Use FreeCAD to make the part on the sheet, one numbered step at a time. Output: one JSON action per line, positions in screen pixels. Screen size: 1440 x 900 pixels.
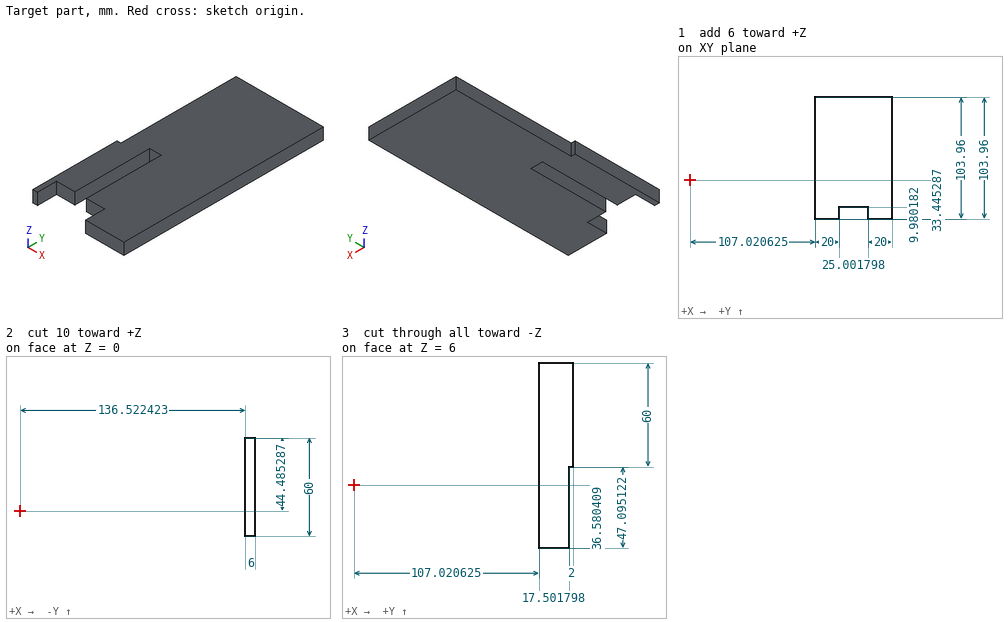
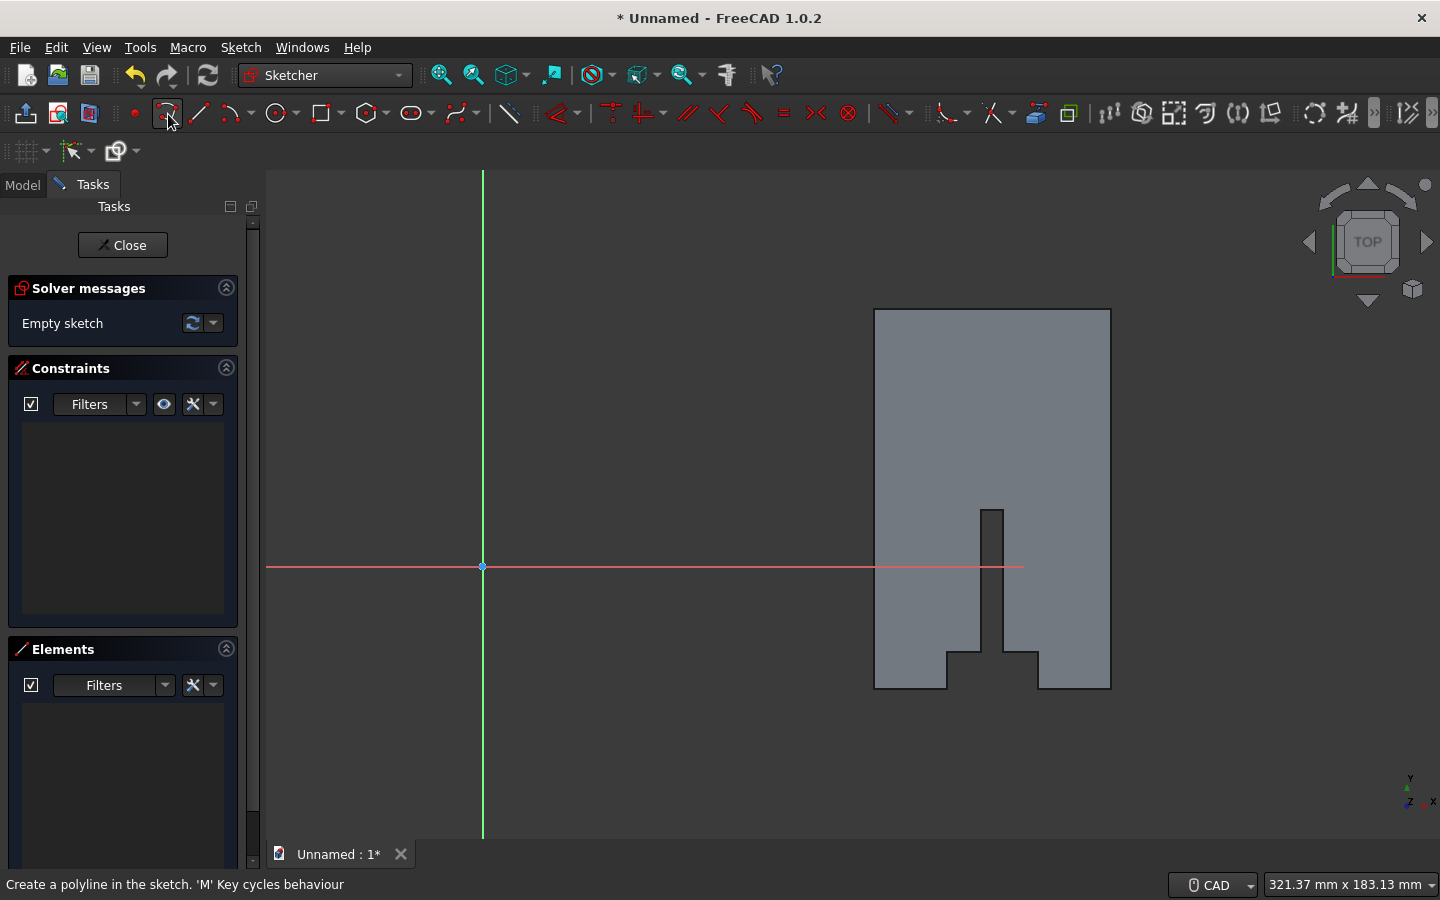
{"action": "left_click", "coordinate": [874, 700]}
{"action": "left_click", "coordinate": [938, 700]}
{"action": "left_click", "coordinate": [938, 528]}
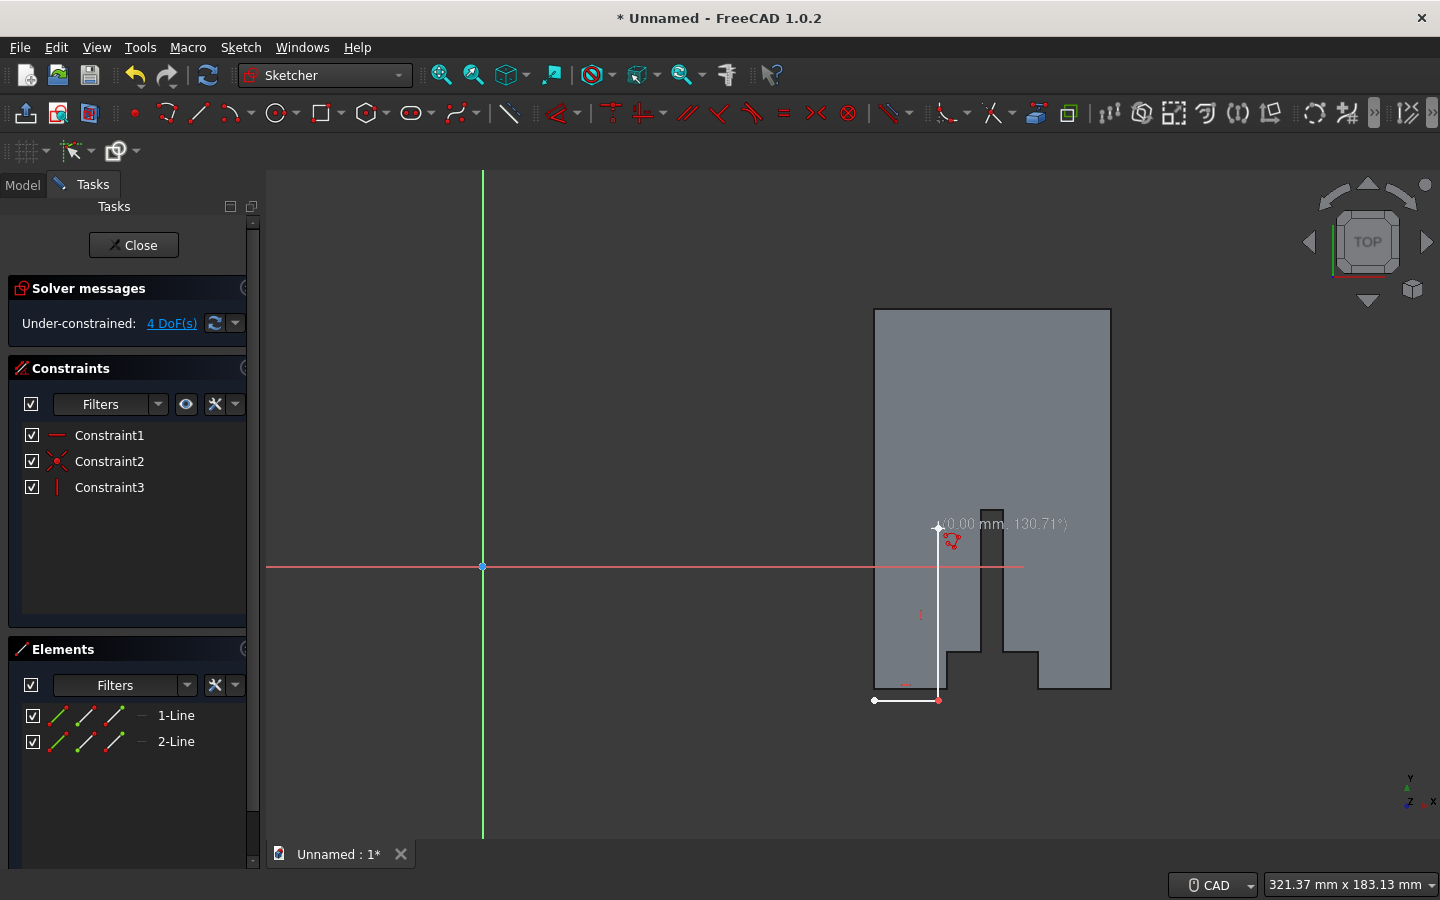
{"action": "scroll", "coordinate": [945, 528], "scroll_direction": "up", "scroll_amount": 4}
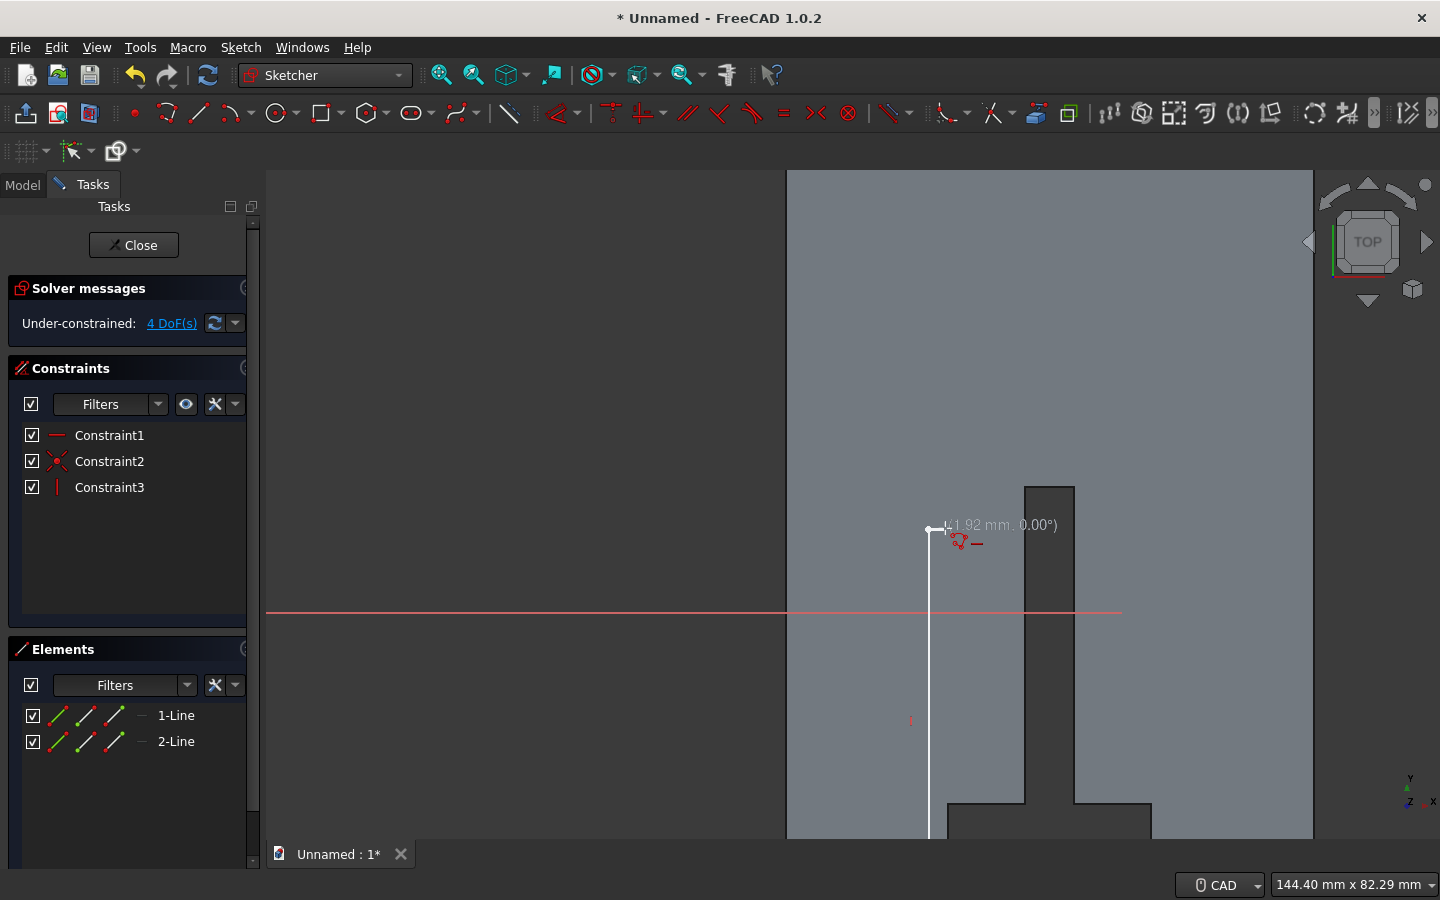
{"action": "left_click", "coordinate": [944, 527]}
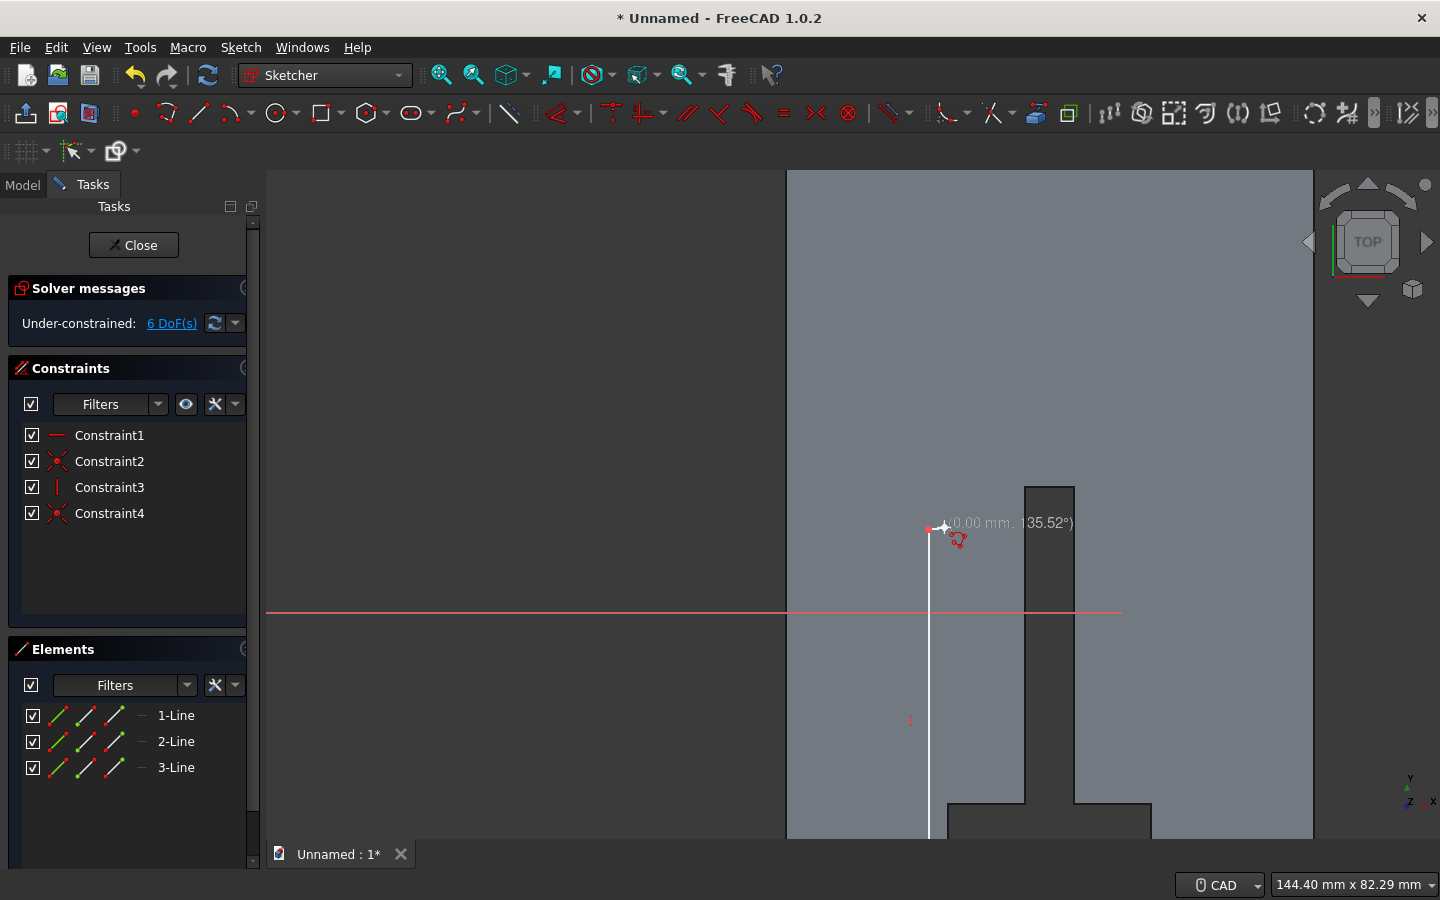
{"action": "scroll", "coordinate": [1216, 540], "scroll_direction": "down", "scroll_amount": 3}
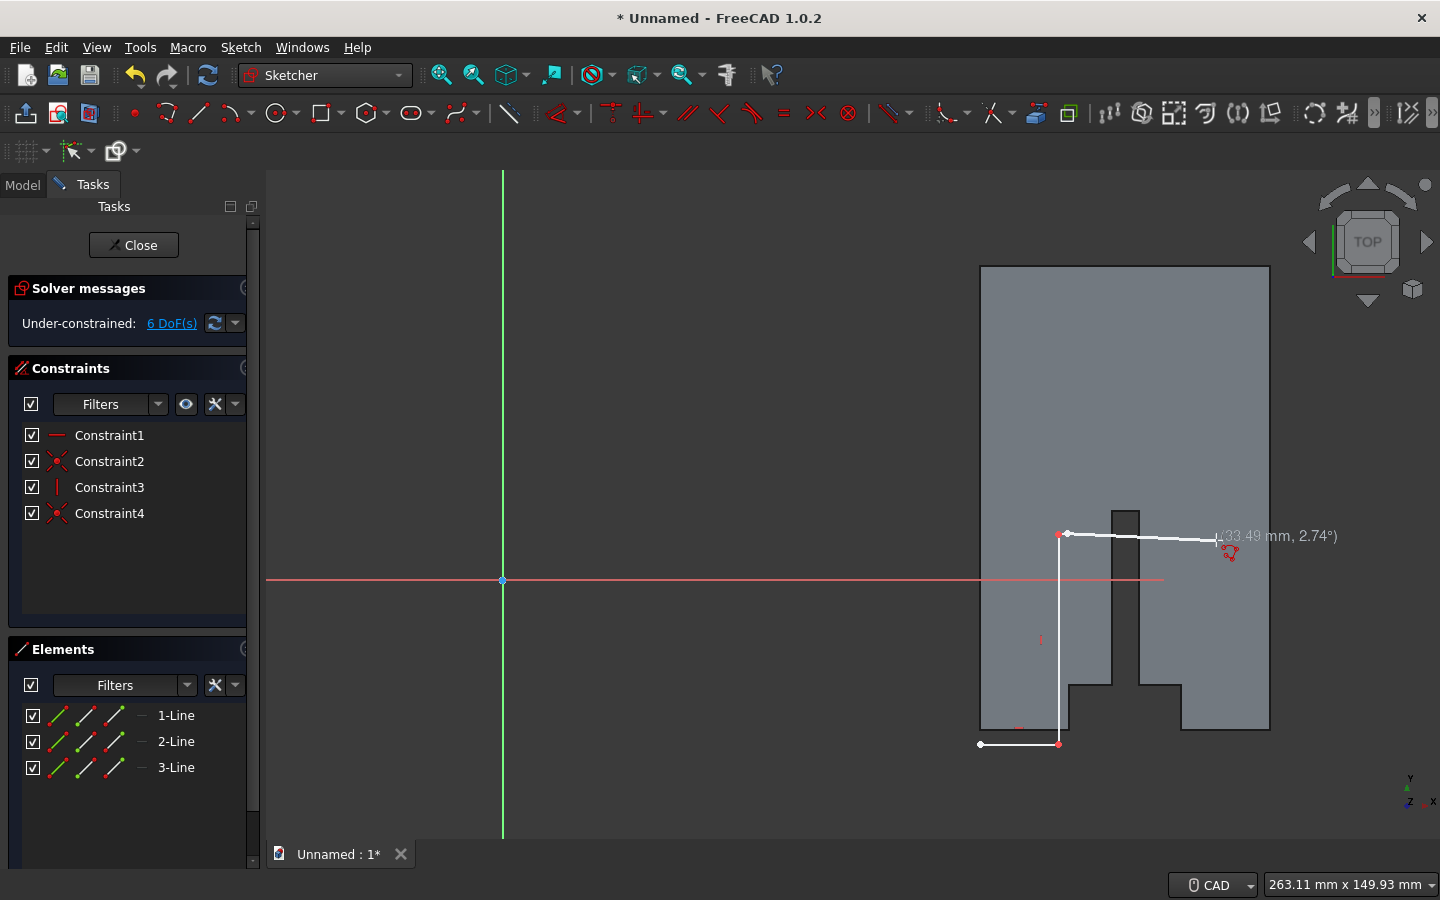
{"action": "left_click", "coordinate": [1067, 266]}
{"action": "left_click", "coordinate": [980, 266]}
{"action": "left_click", "coordinate": [981, 745]}
{"action": "key", "text": "Escape"}
{"action": "key", "text": "Escape"}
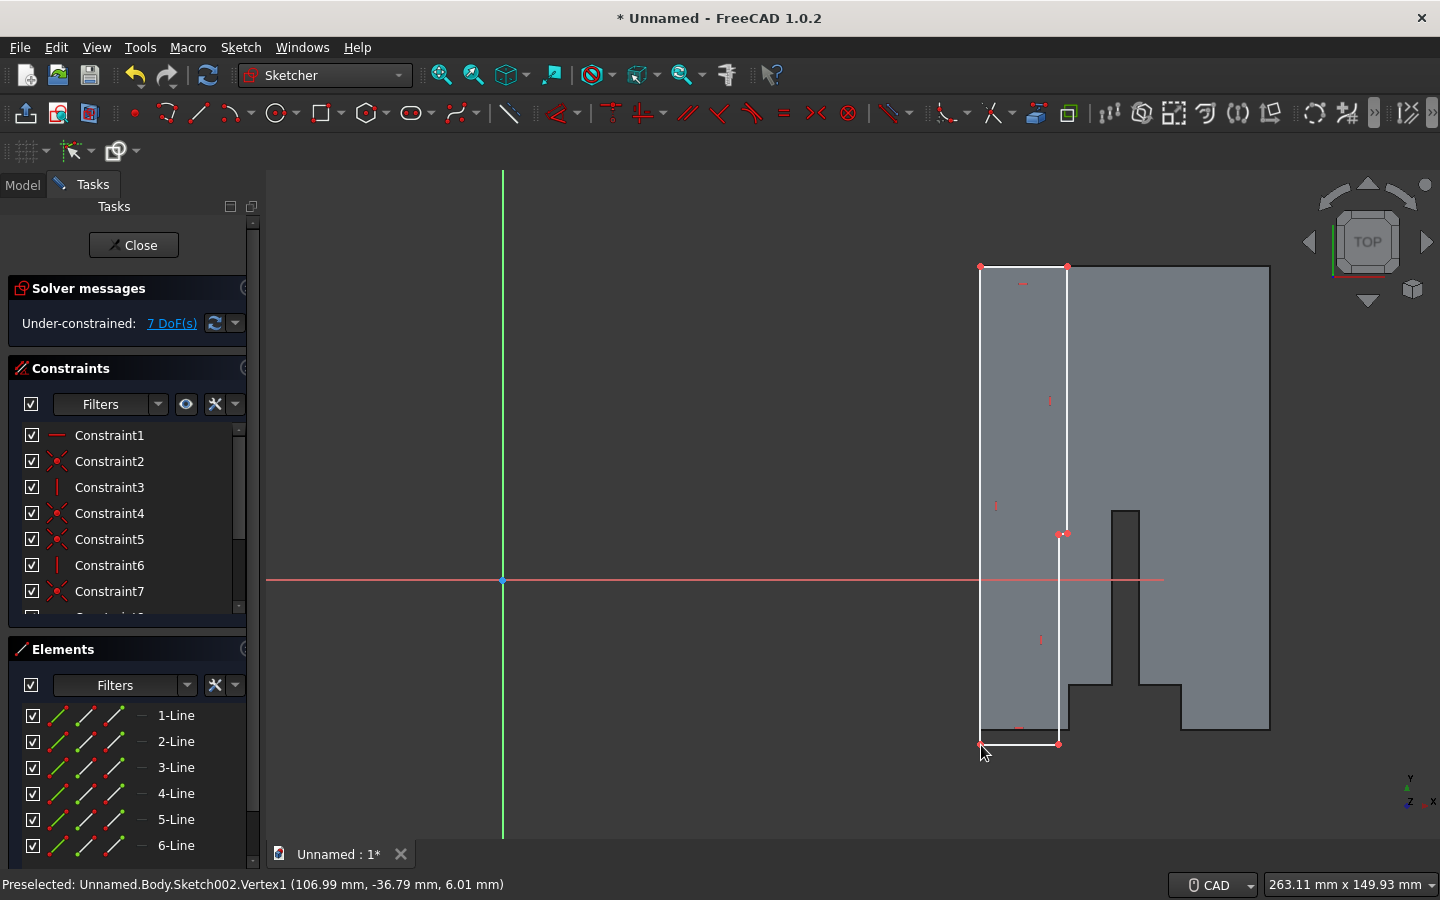
{"action": "scroll", "coordinate": [1063, 534], "scroll_direction": "up", "scroll_amount": 6}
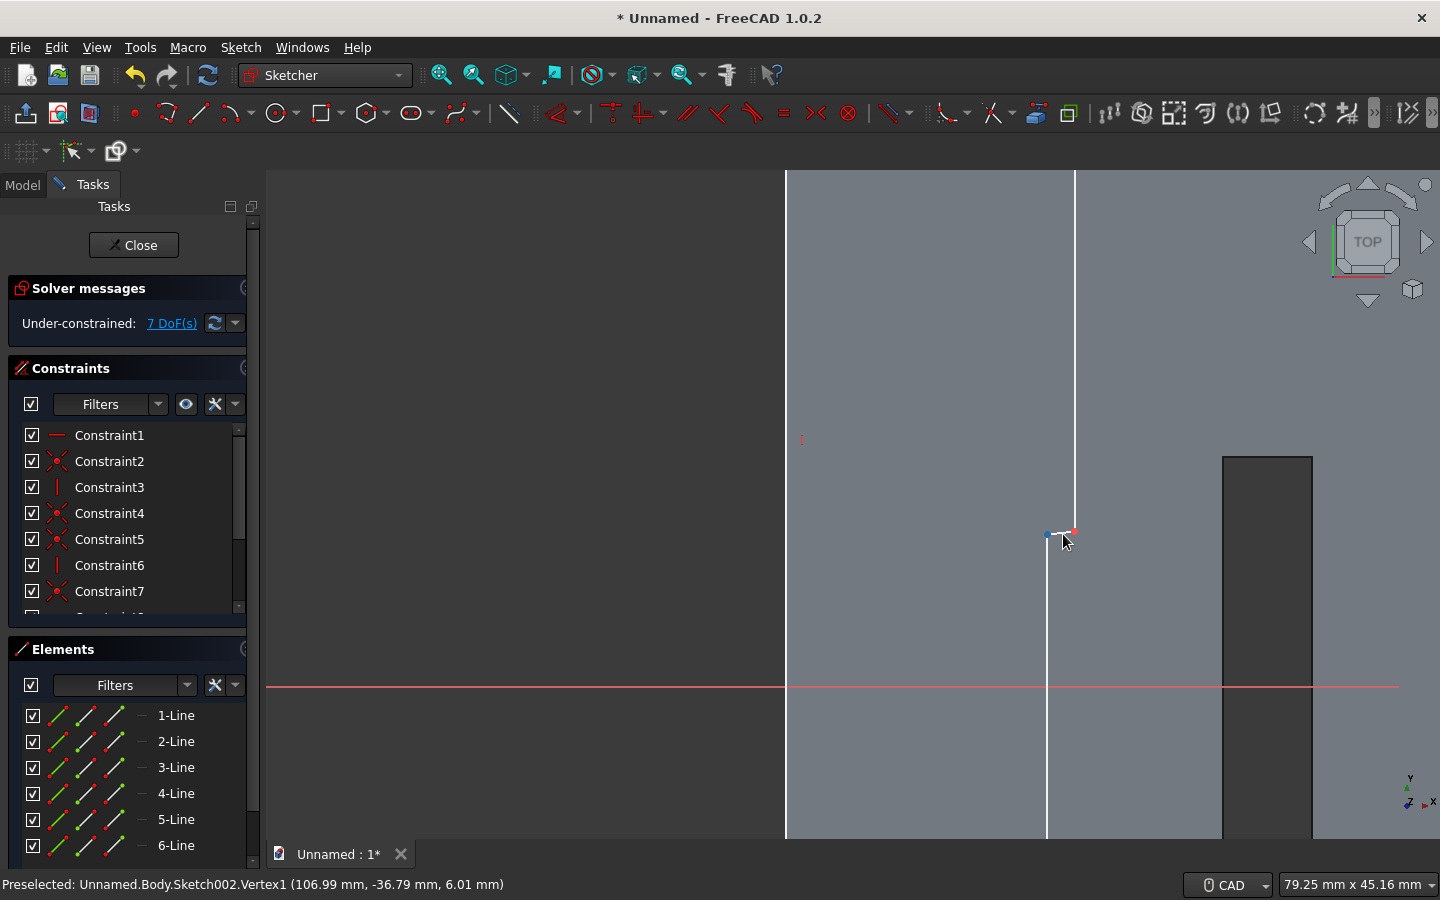
{"action": "left_click", "coordinate": [1061, 533]}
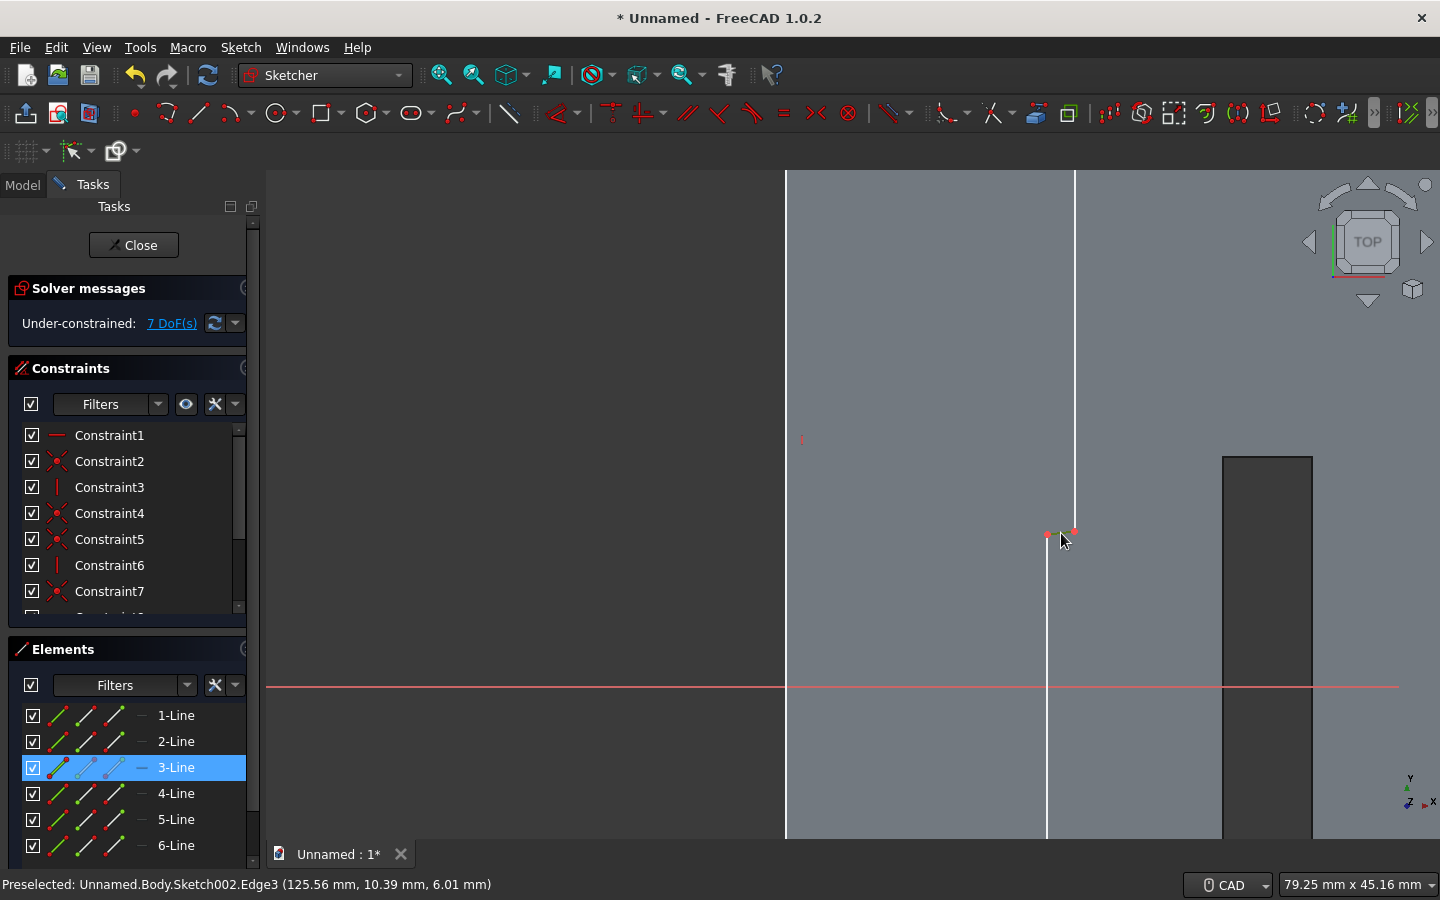
{"action": "key", "text": "h"}